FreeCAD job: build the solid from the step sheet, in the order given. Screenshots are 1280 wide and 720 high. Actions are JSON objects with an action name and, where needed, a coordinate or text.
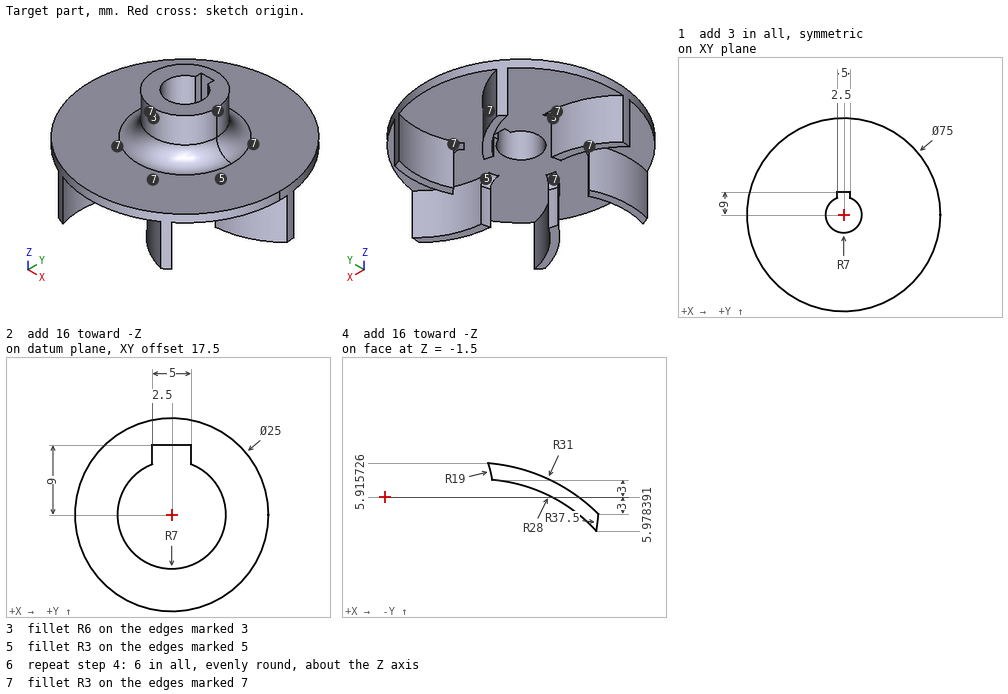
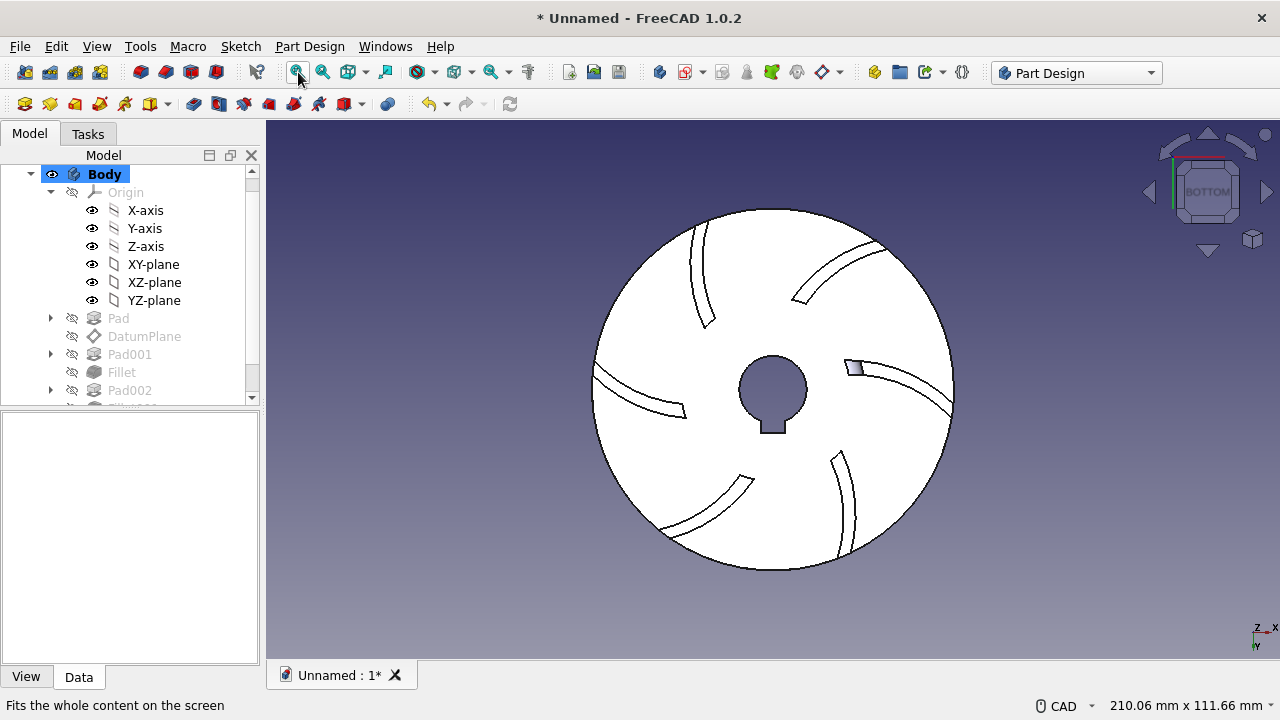
{"action": "scroll", "coordinate": [836, 455], "scroll_direction": "up", "scroll_amount": 6}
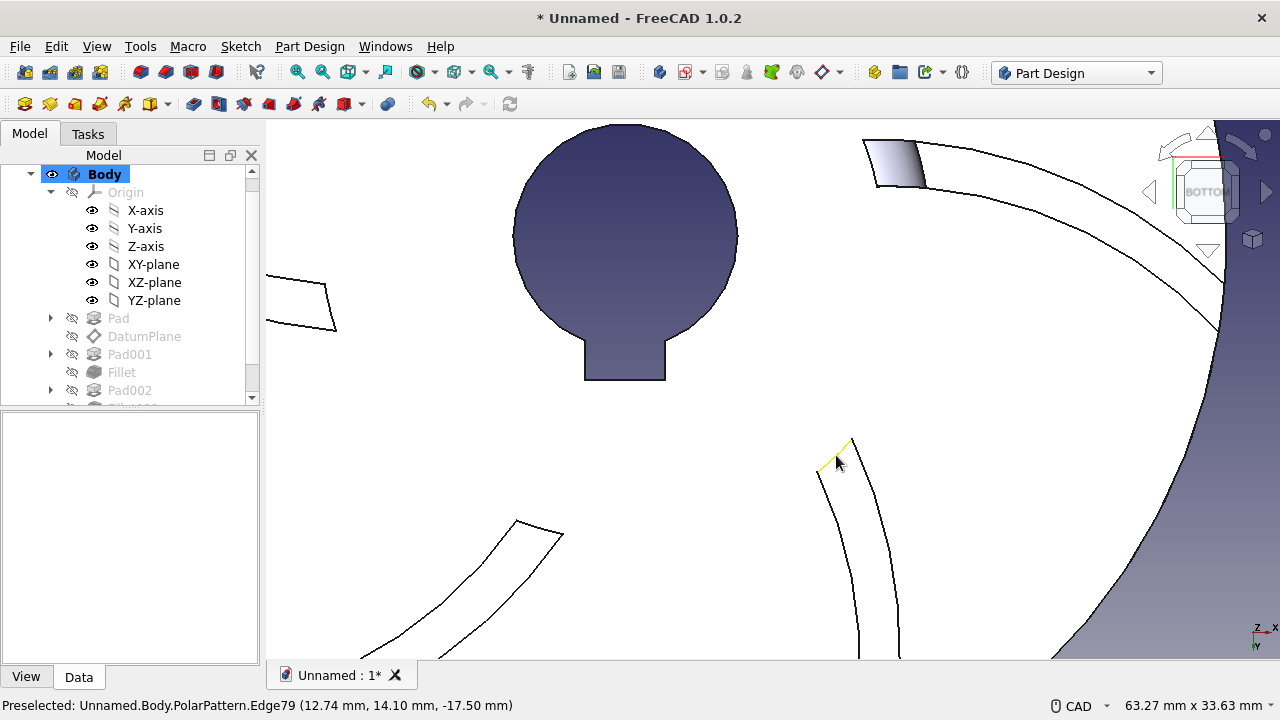
{"action": "left_click", "coordinate": [298, 72]}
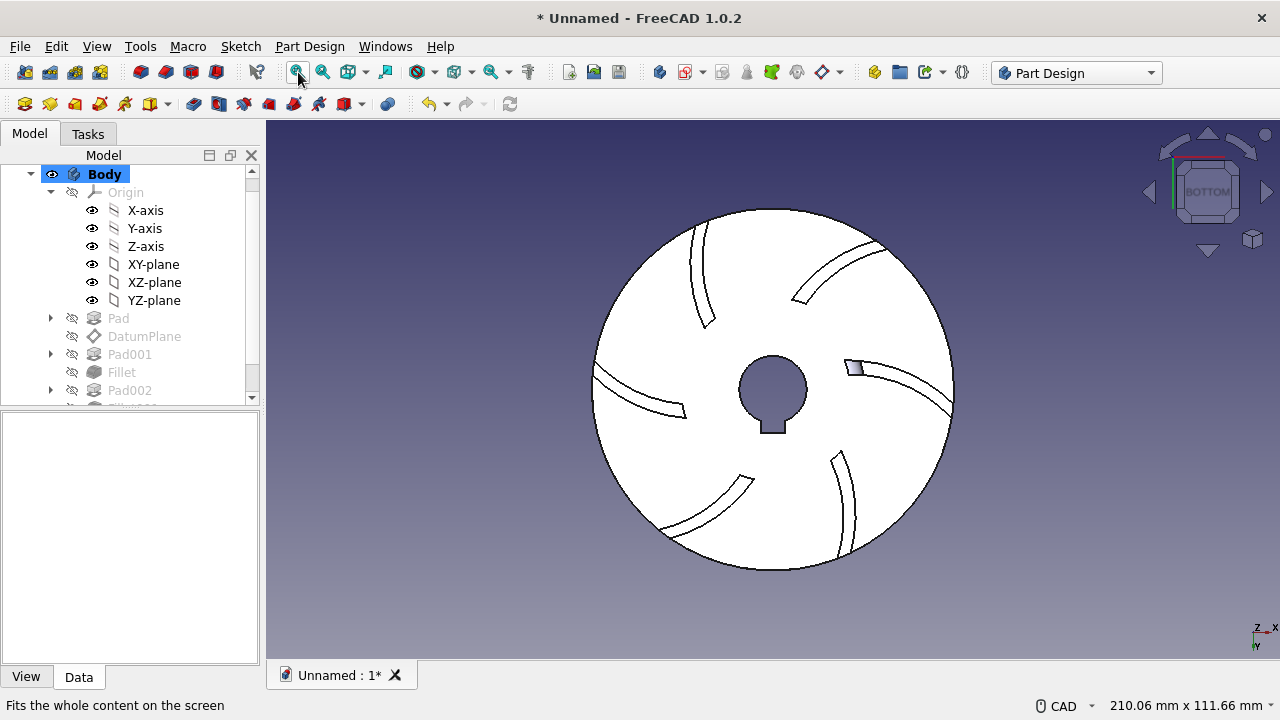
{"action": "key", "text": "4"}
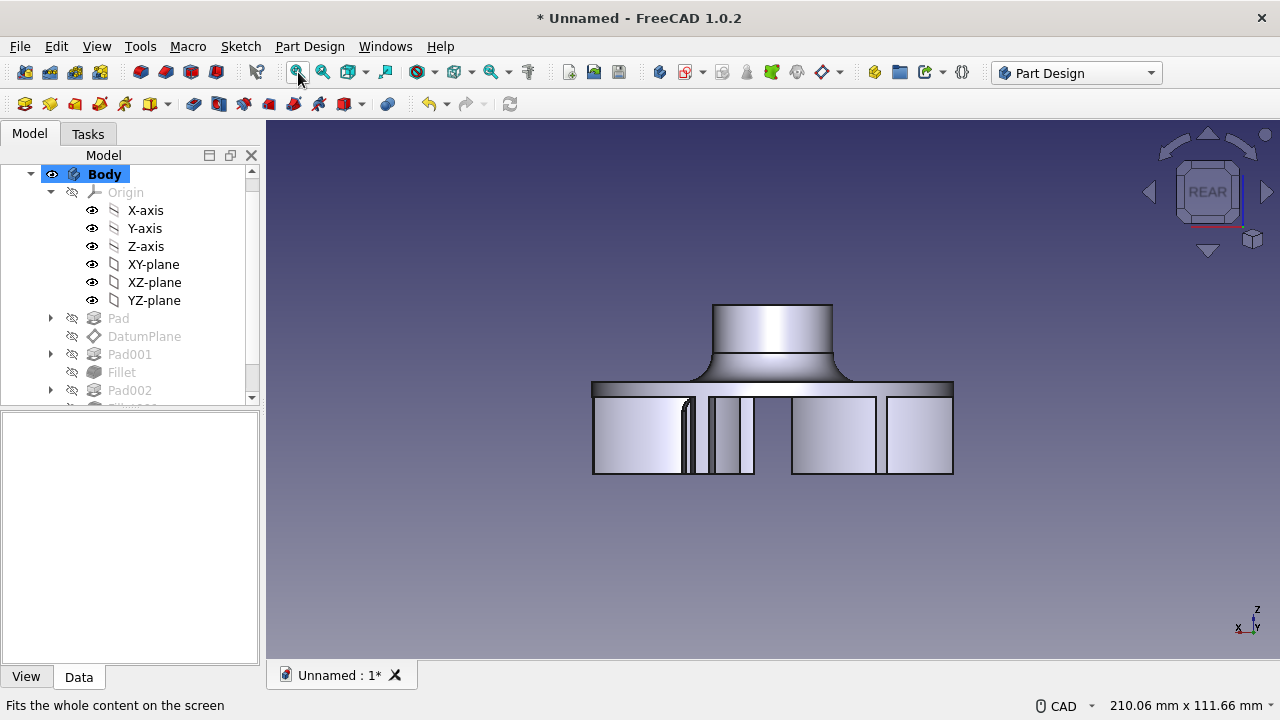
{"action": "left_click", "coordinate": [298, 72]}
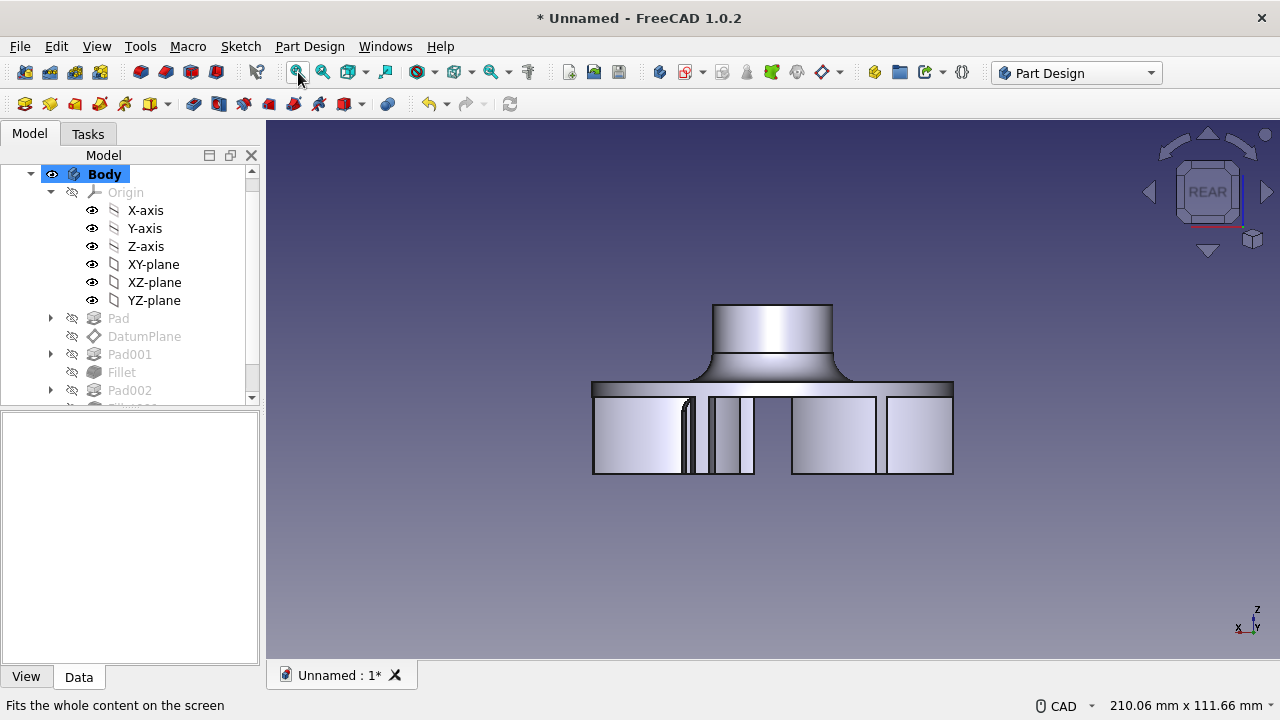
{"action": "scroll", "coordinate": [710, 396], "scroll_direction": "up", "scroll_amount": 6}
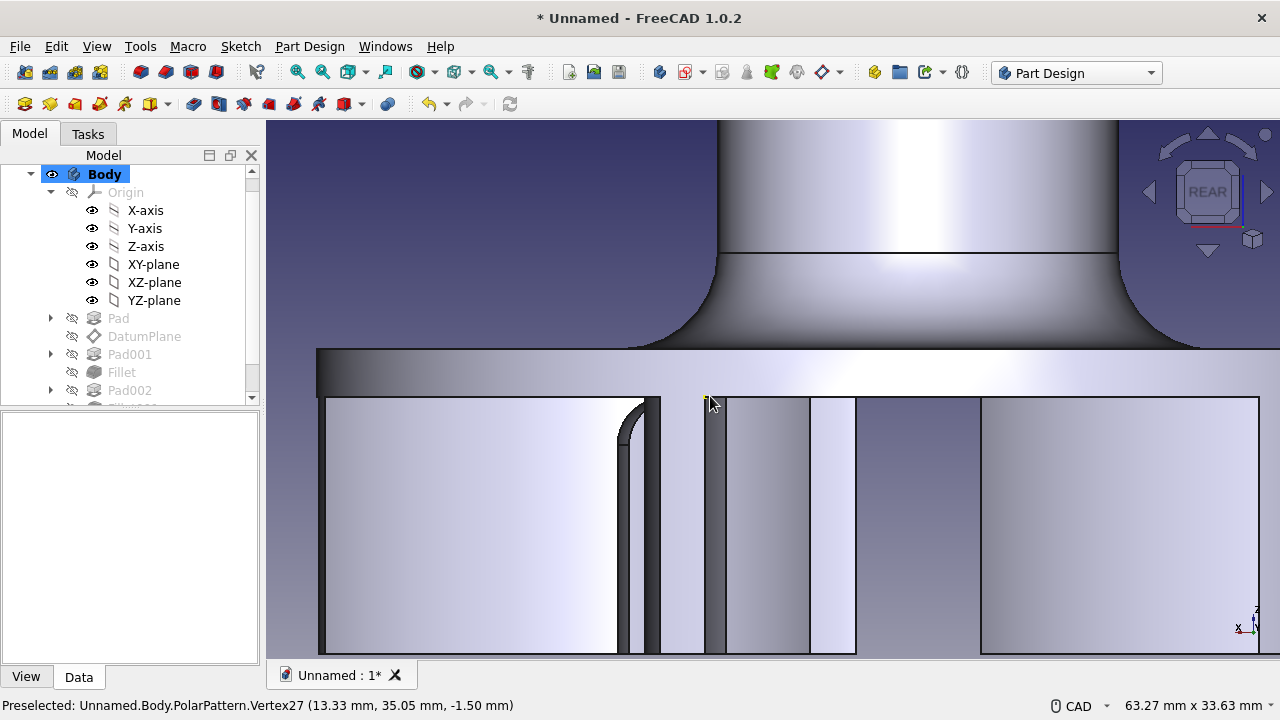
{"action": "left_click", "coordinate": [298, 72]}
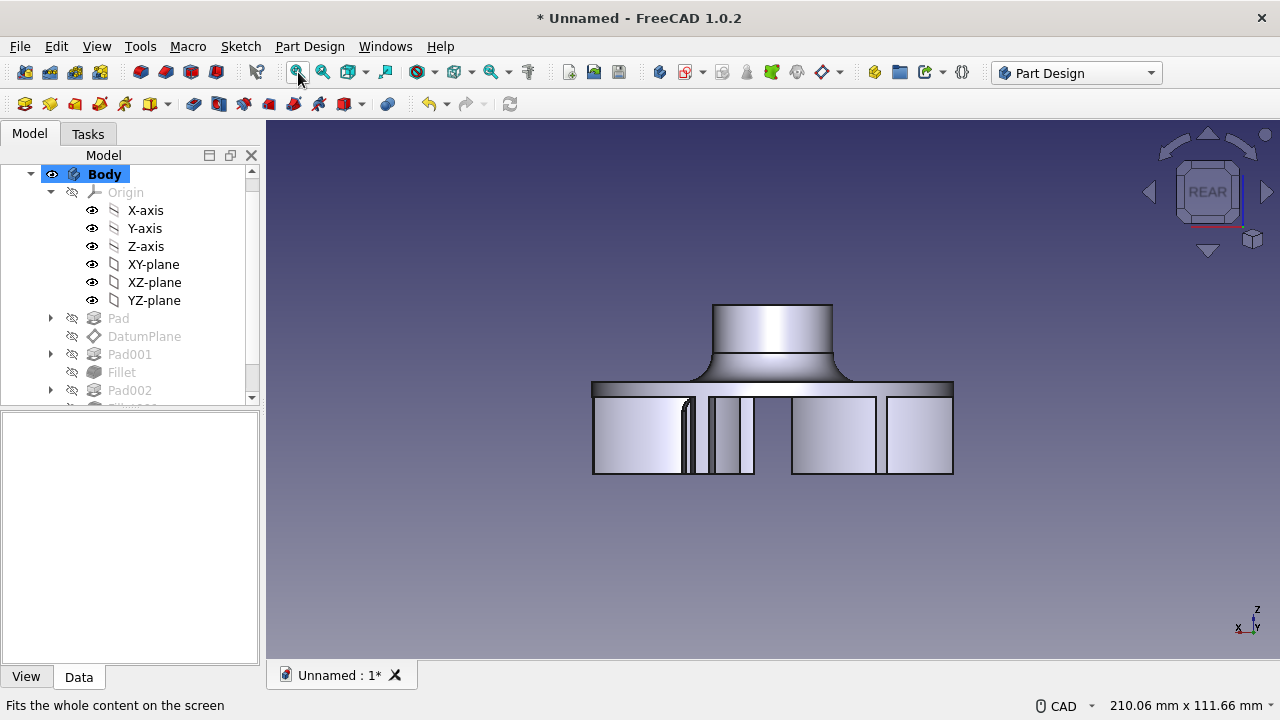
{"action": "key", "text": "6"}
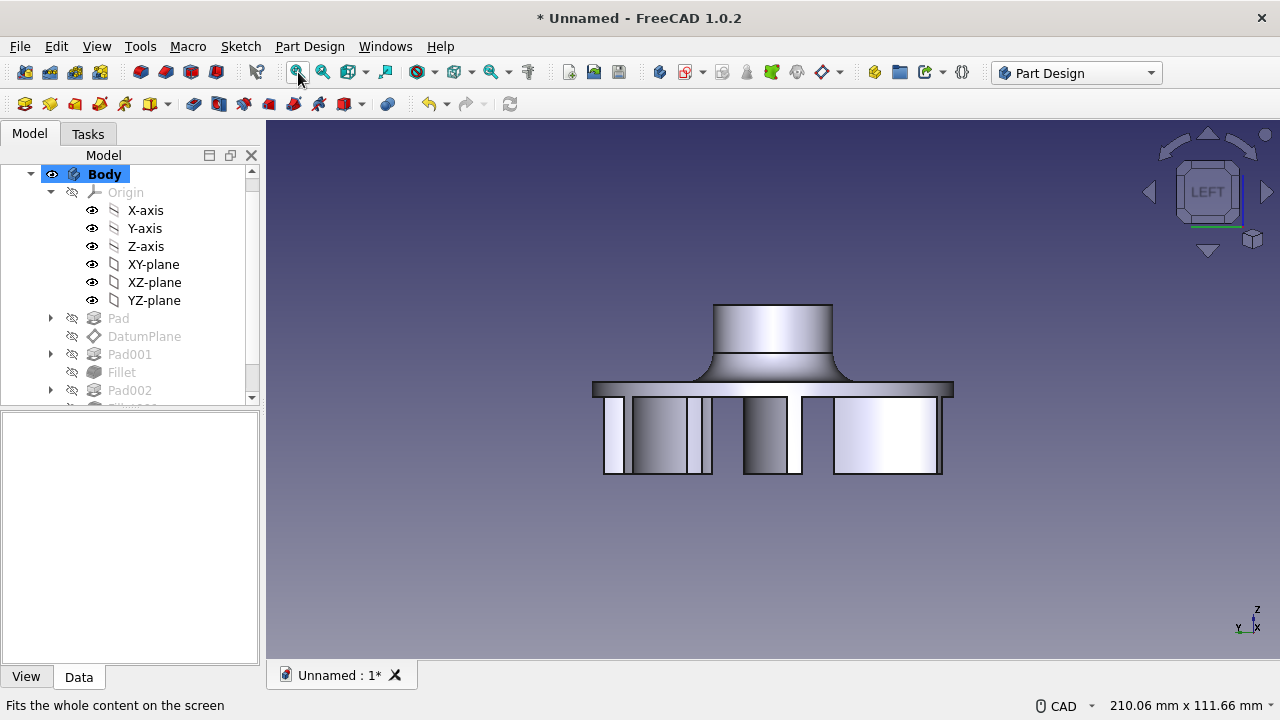
{"action": "left_click", "coordinate": [298, 72]}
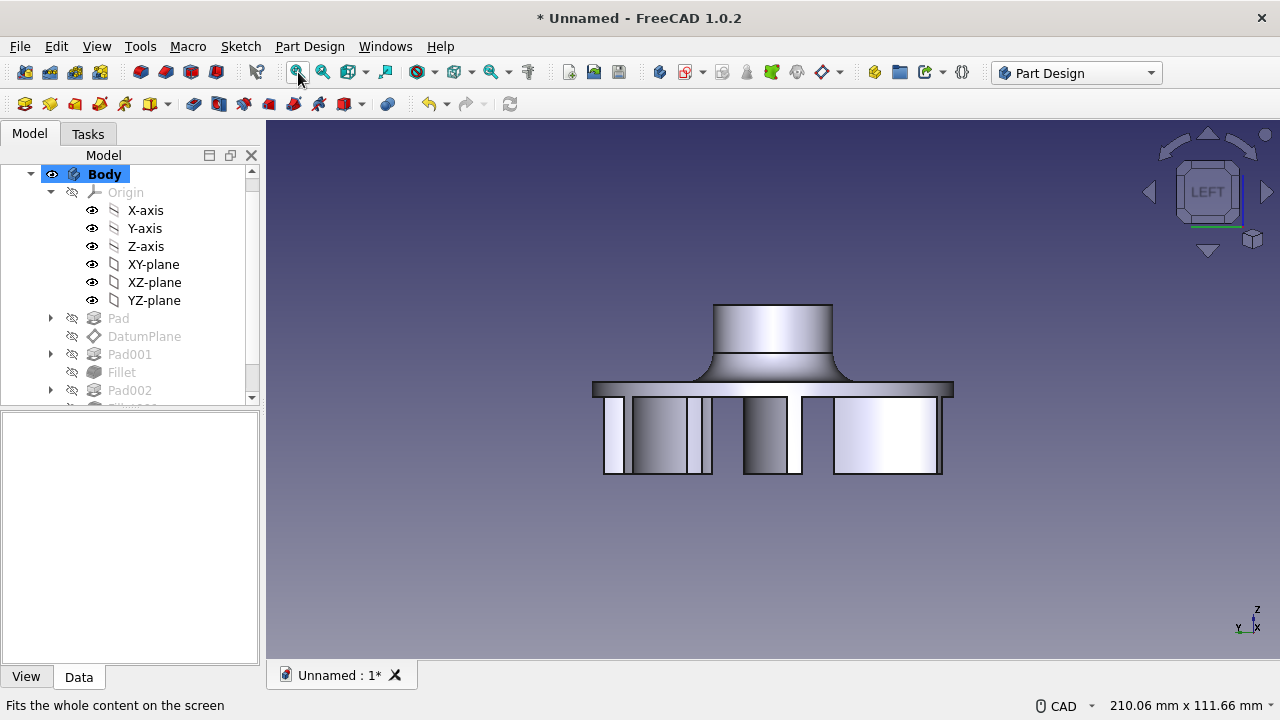
{"action": "scroll", "coordinate": [707, 396], "scroll_direction": "up", "scroll_amount": 6}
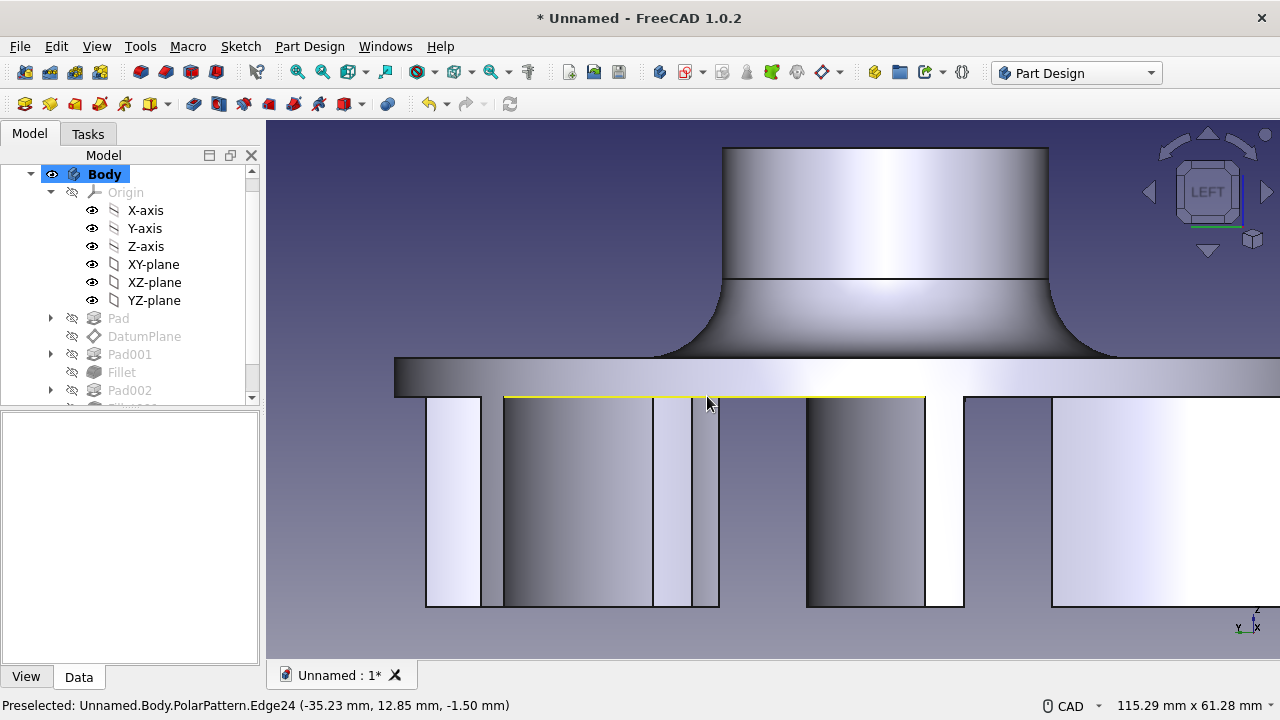
{"action": "left_click", "coordinate": [298, 72]}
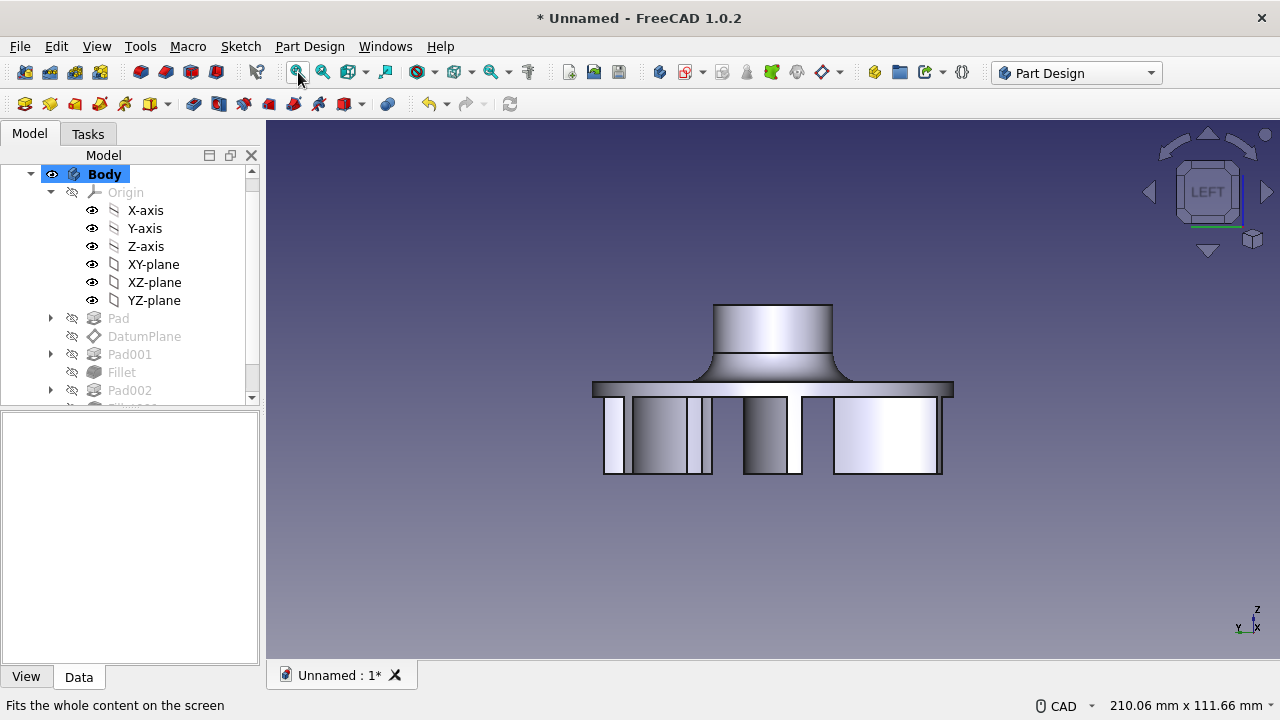
{"action": "key", "text": "v 3"}